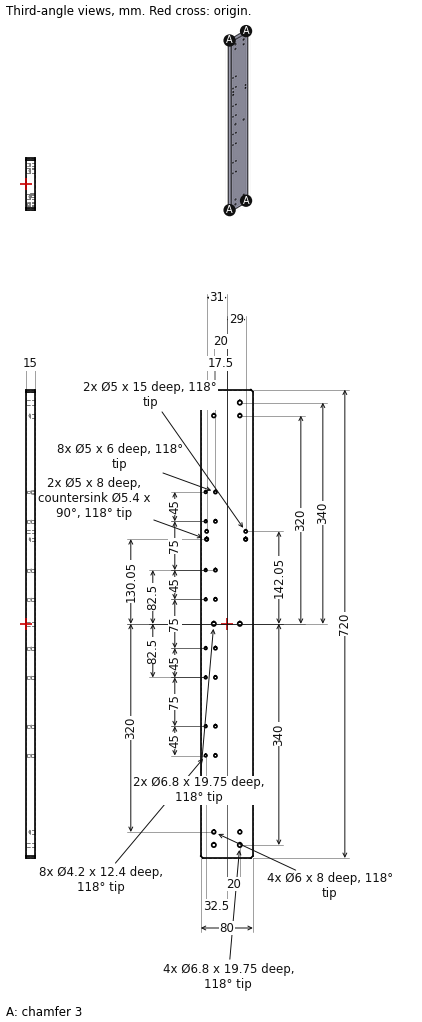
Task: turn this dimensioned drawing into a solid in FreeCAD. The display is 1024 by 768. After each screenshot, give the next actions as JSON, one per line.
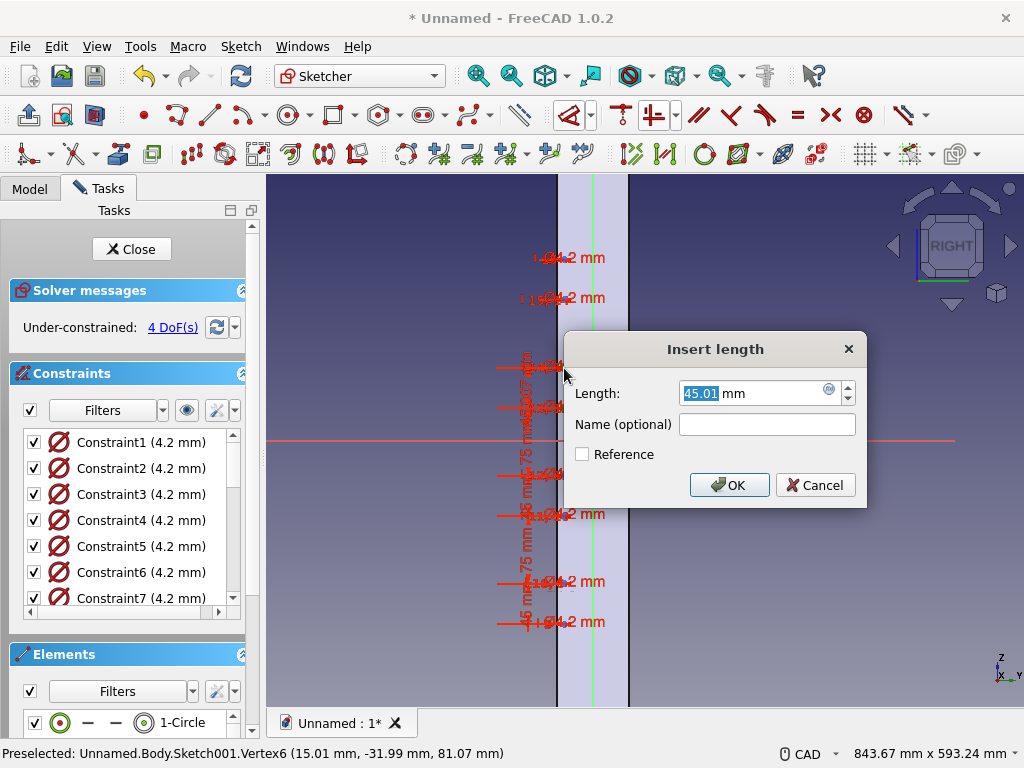
{"action": "type", "text": "45"}
{"action": "key", "text": "Return"}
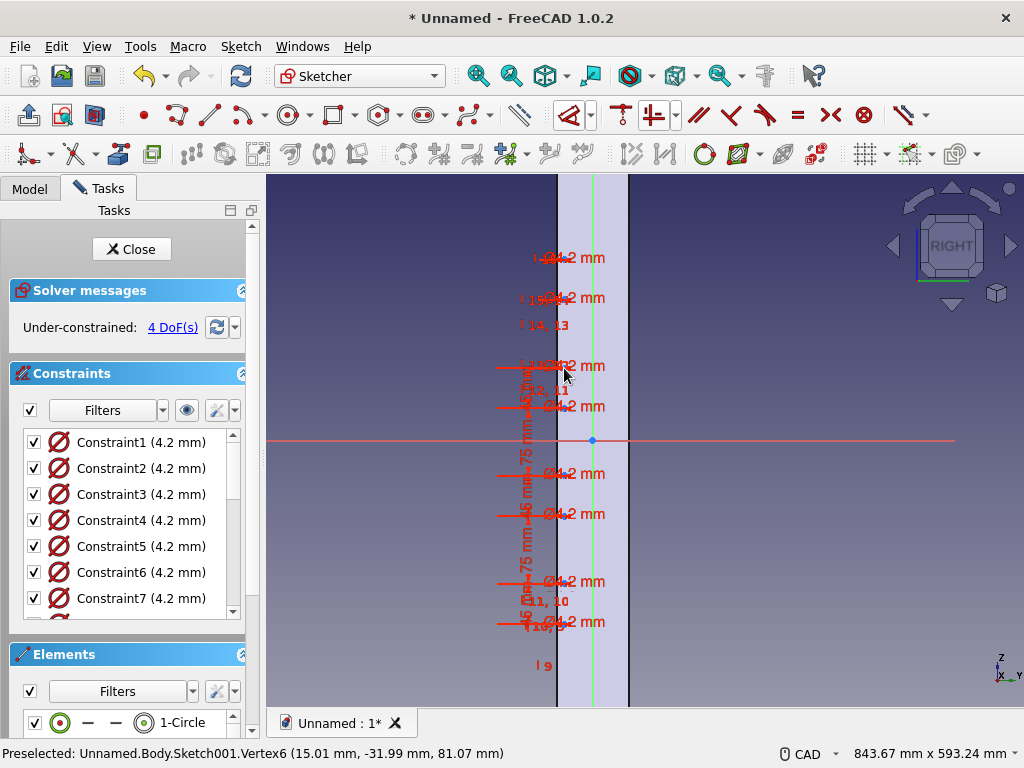
{"action": "left_click", "coordinate": [564, 368]}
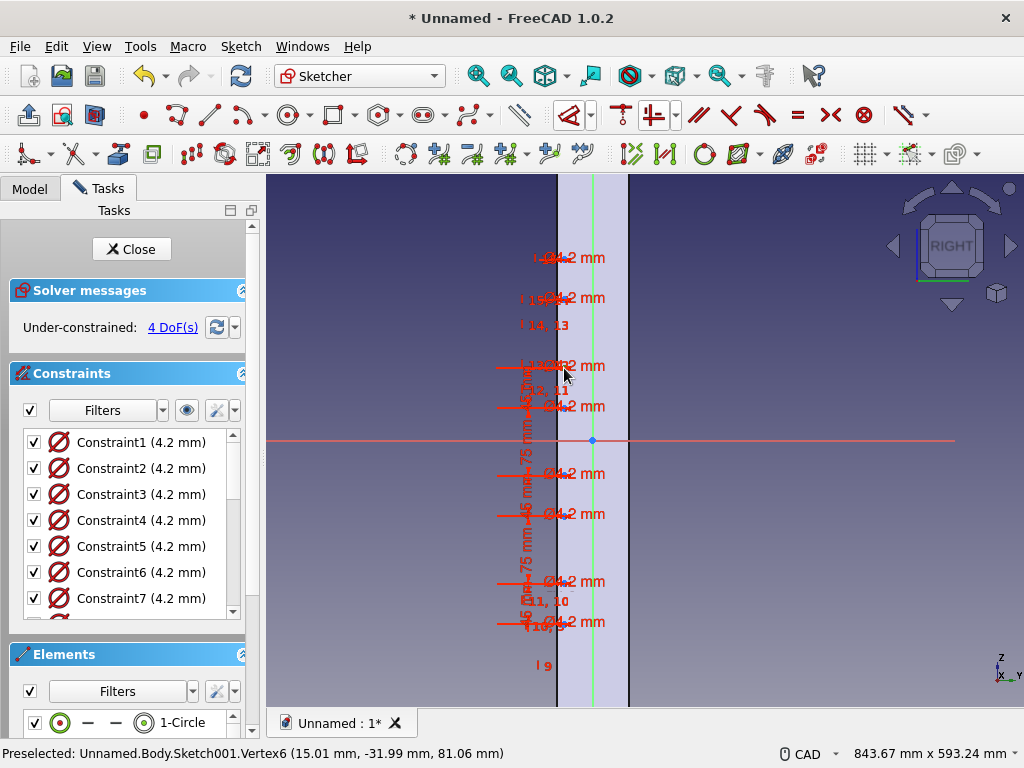
{"action": "left_click", "coordinate": [564, 300]}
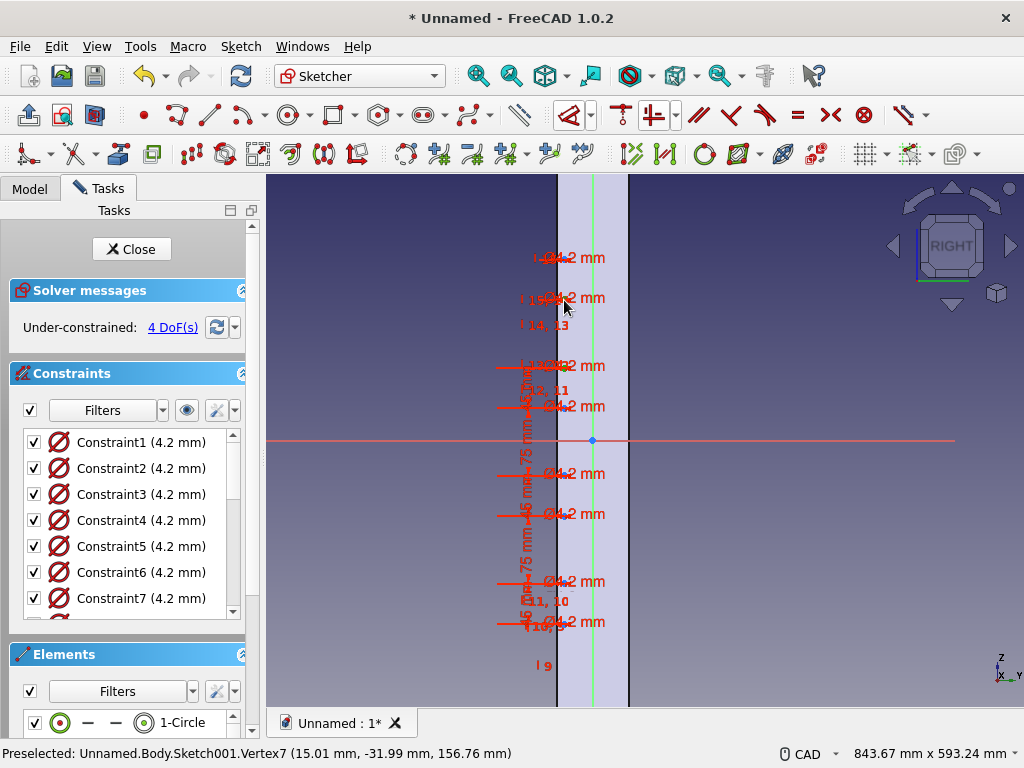
{"action": "left_click", "coordinate": [590, 116]}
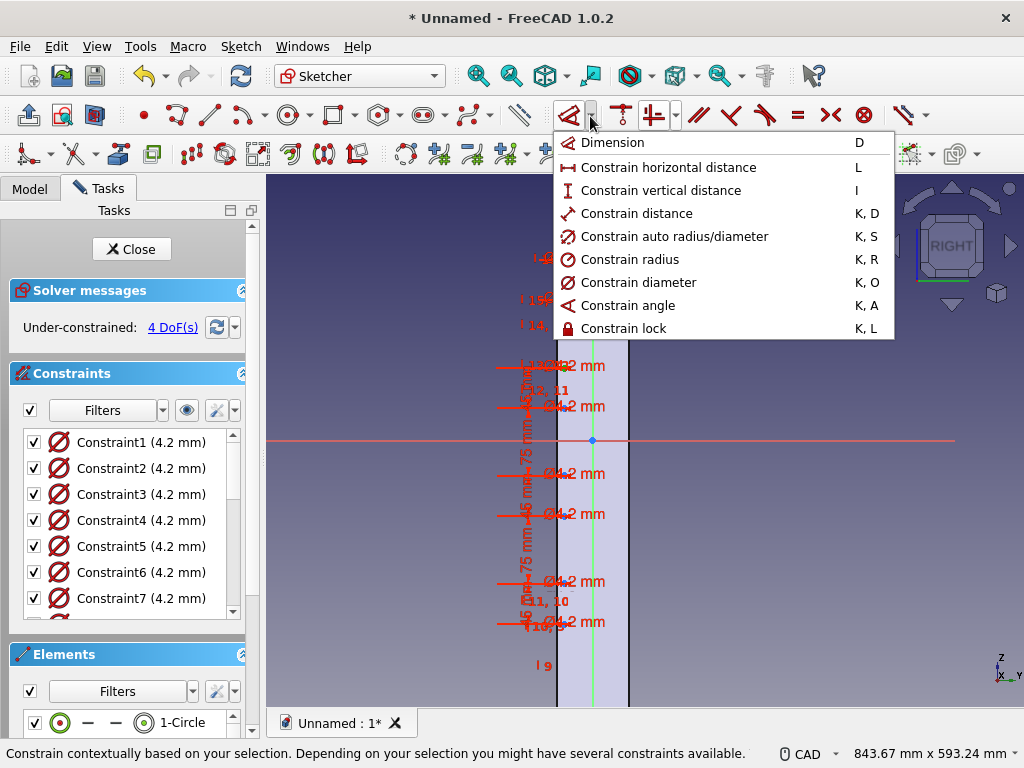
{"action": "left_click", "coordinate": [724, 190]}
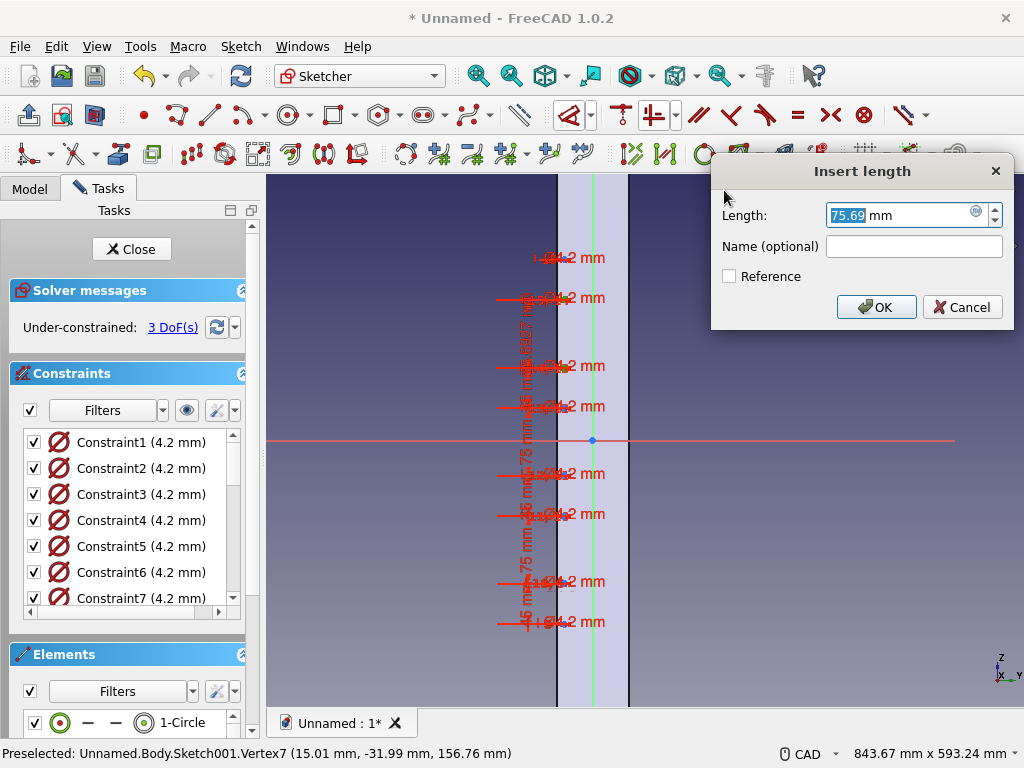
{"action": "type", "text": "75"}
{"action": "key", "text": "Return"}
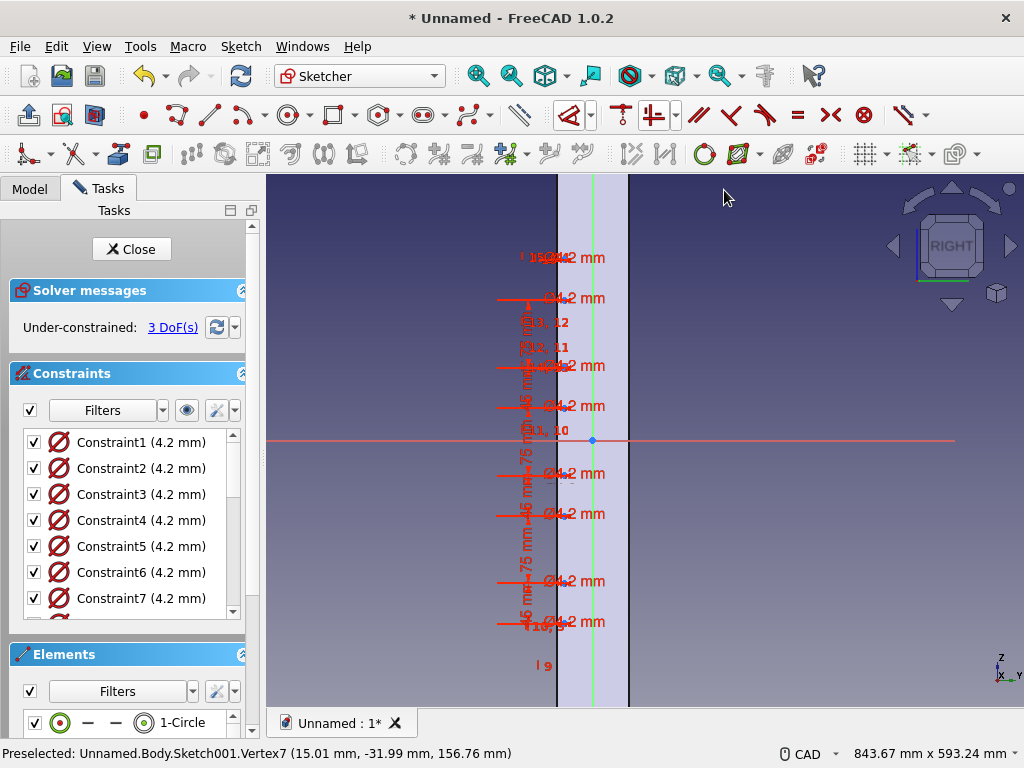
{"action": "left_click", "coordinate": [564, 300]}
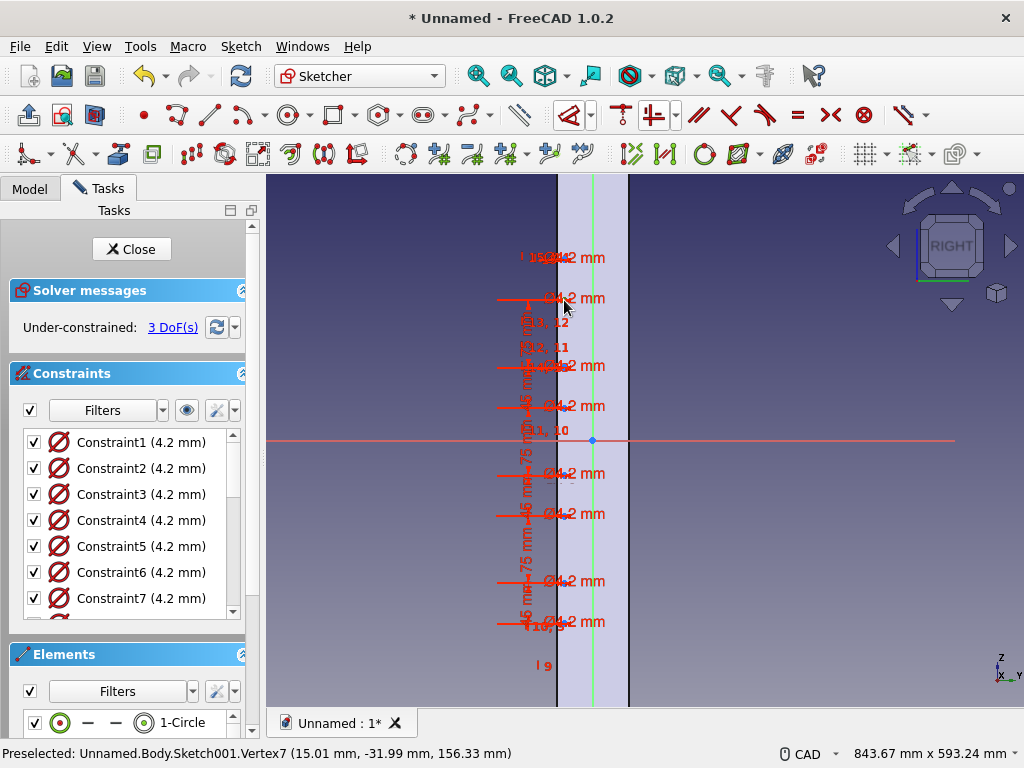
{"action": "left_click", "coordinate": [564, 260]}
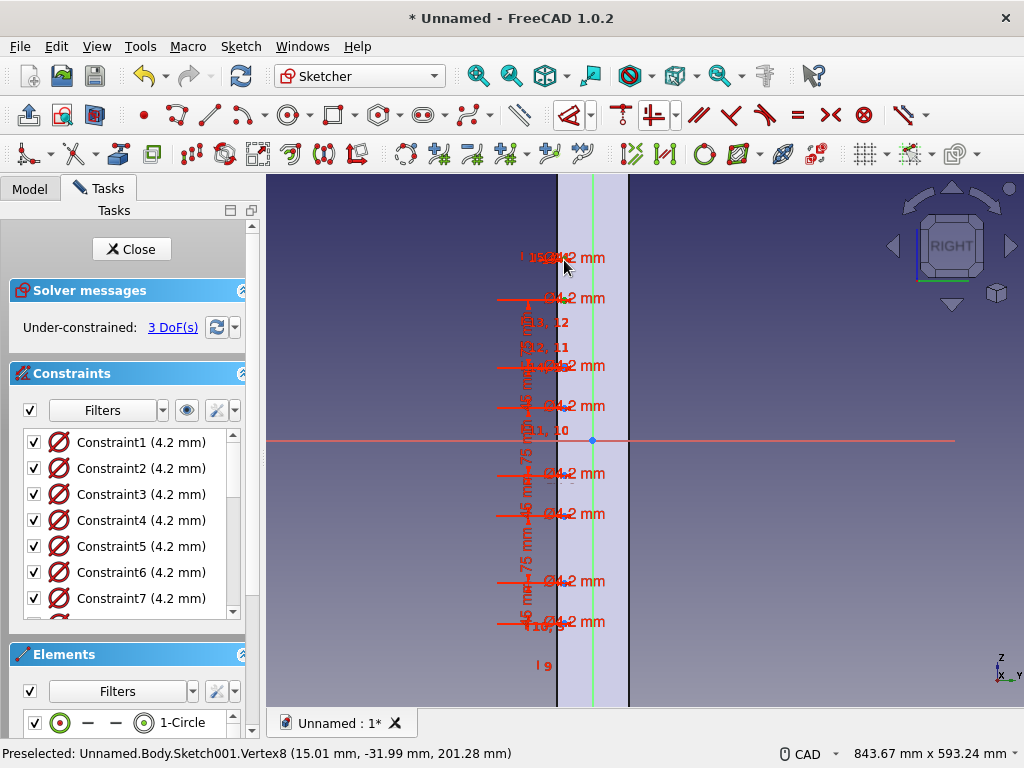
{"action": "left_click", "coordinate": [590, 116]}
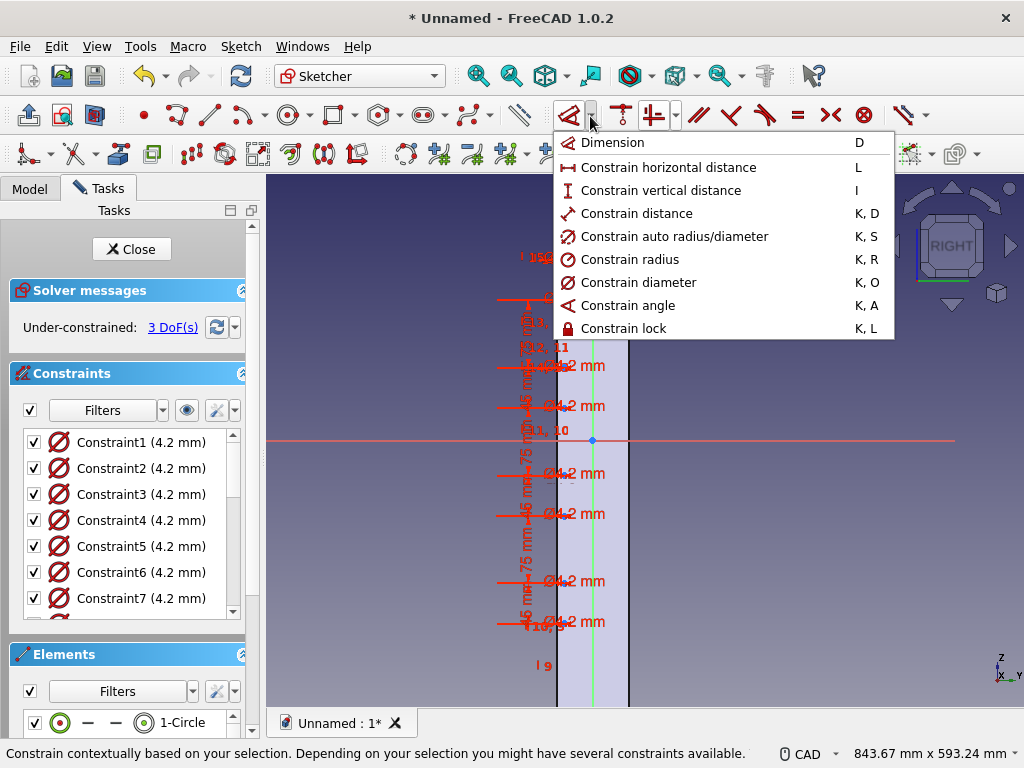
{"action": "left_click", "coordinate": [724, 190]}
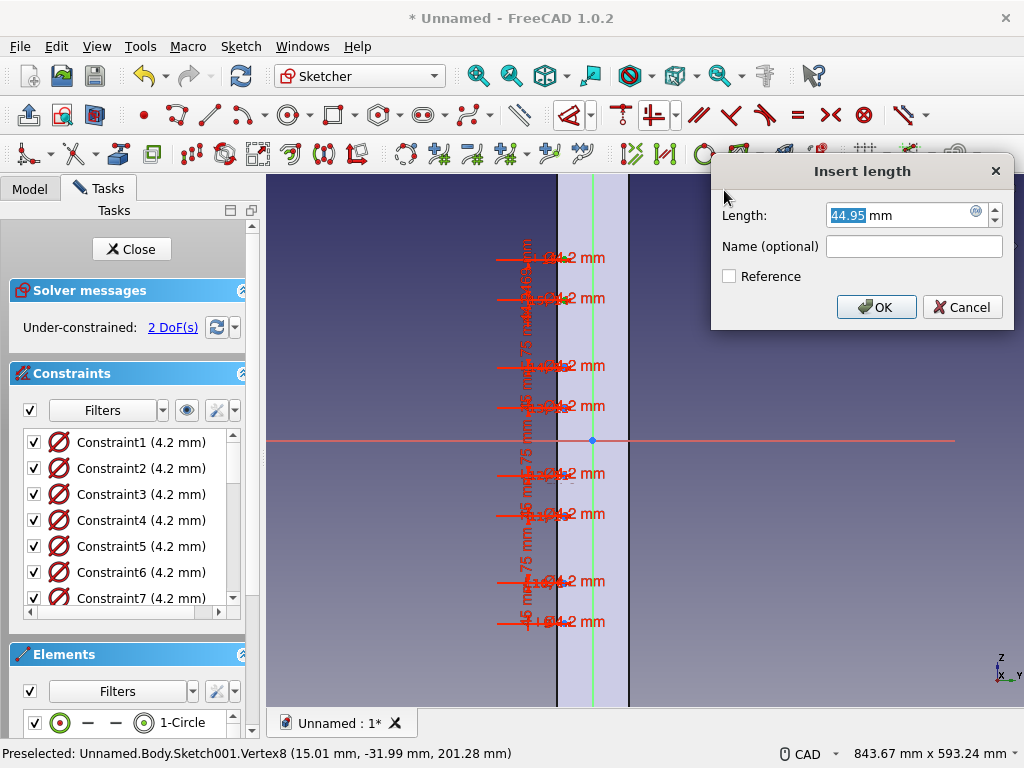
{"action": "type", "text": "45"}
{"action": "key", "text": "Return"}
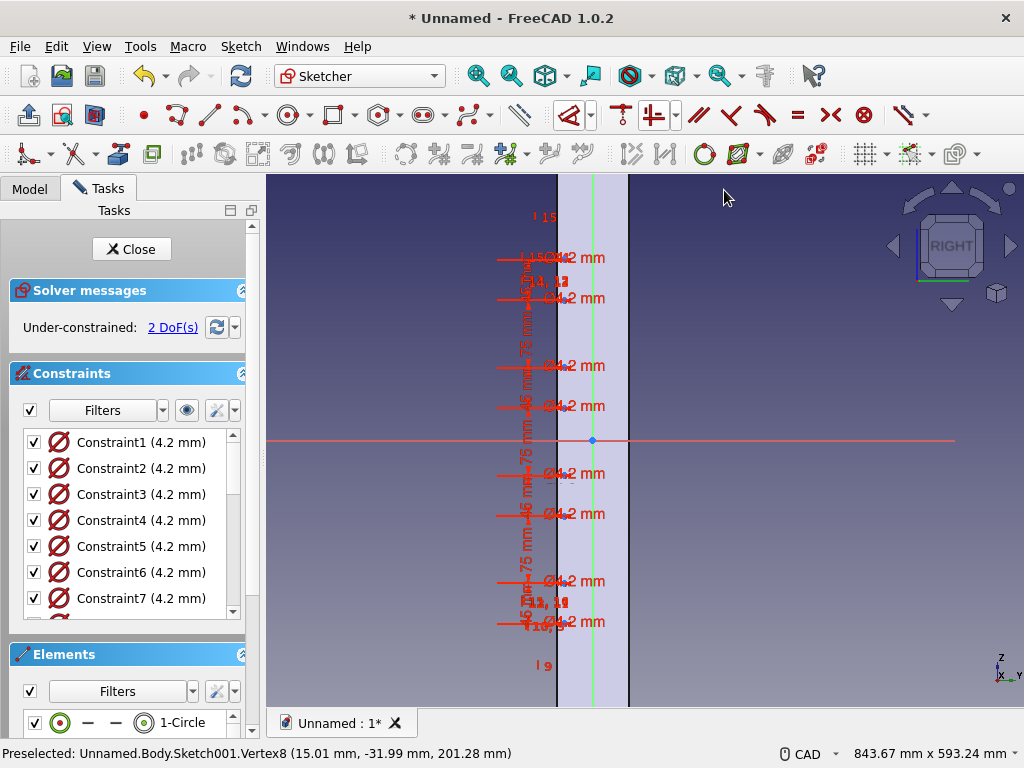
{"action": "scroll", "coordinate": [564, 624], "scroll_direction": "up", "scroll_amount": 2}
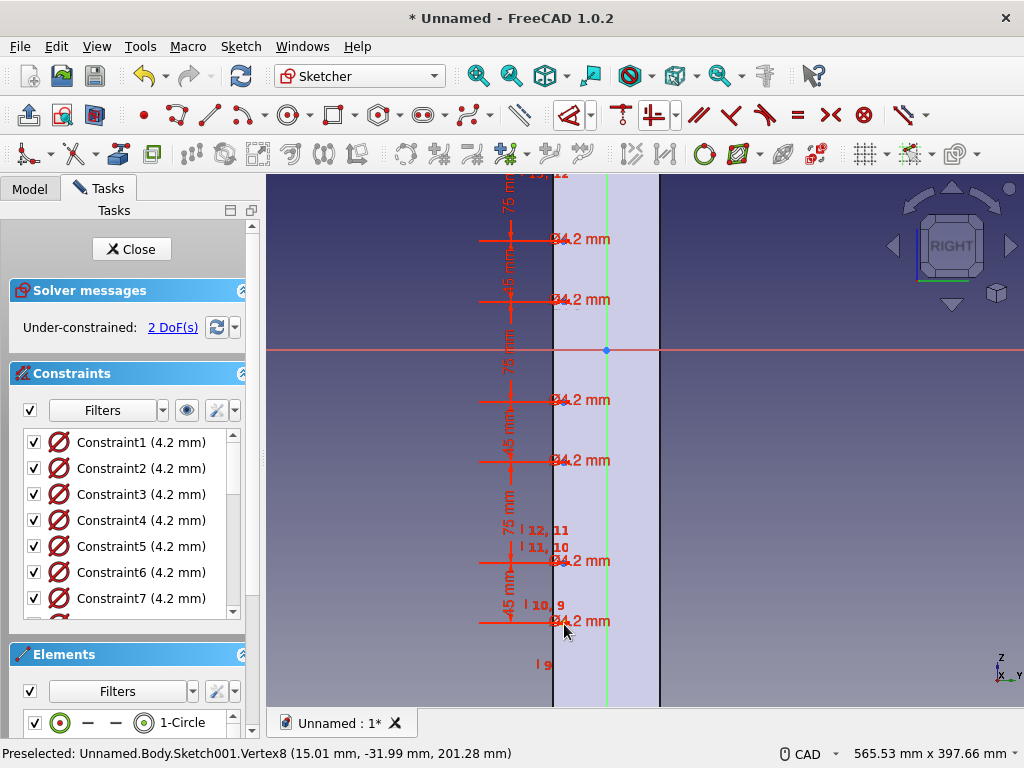
{"action": "left_click", "coordinate": [564, 623]}